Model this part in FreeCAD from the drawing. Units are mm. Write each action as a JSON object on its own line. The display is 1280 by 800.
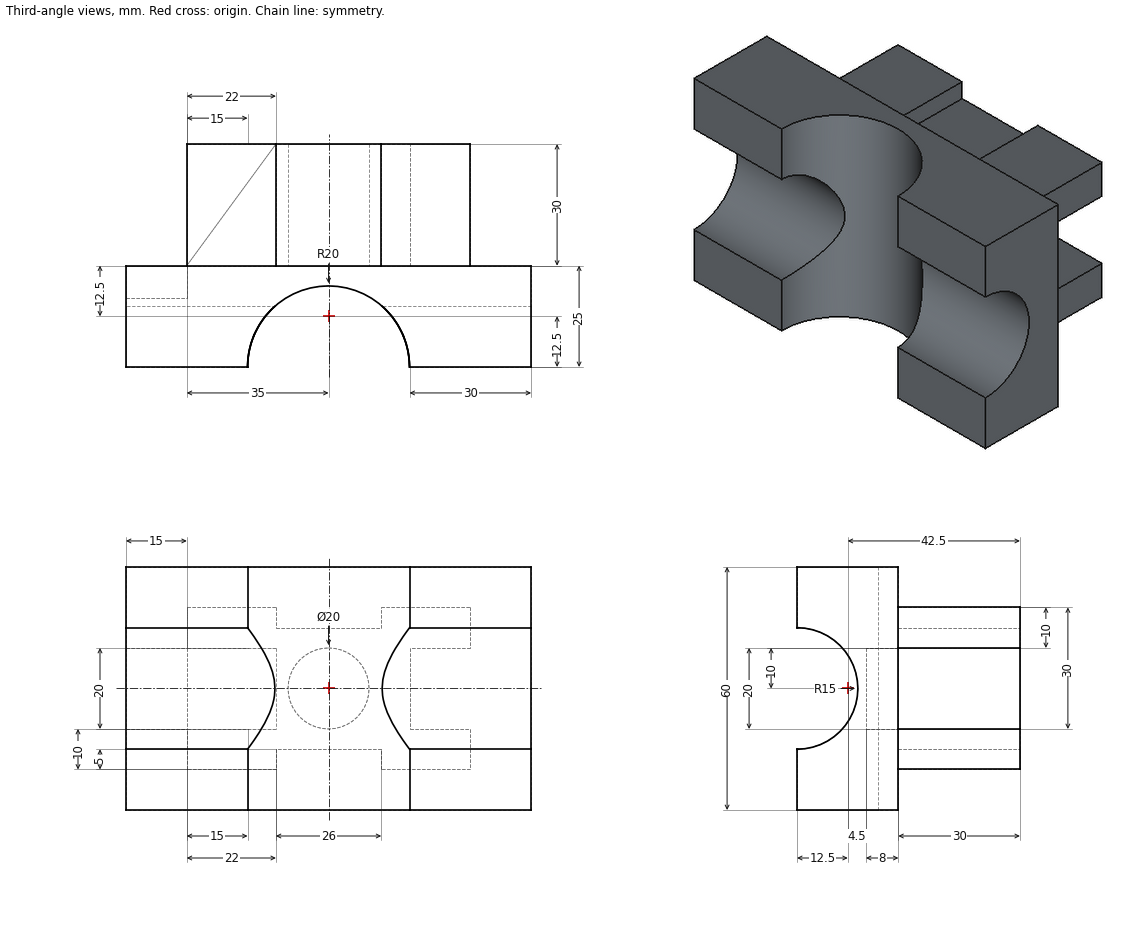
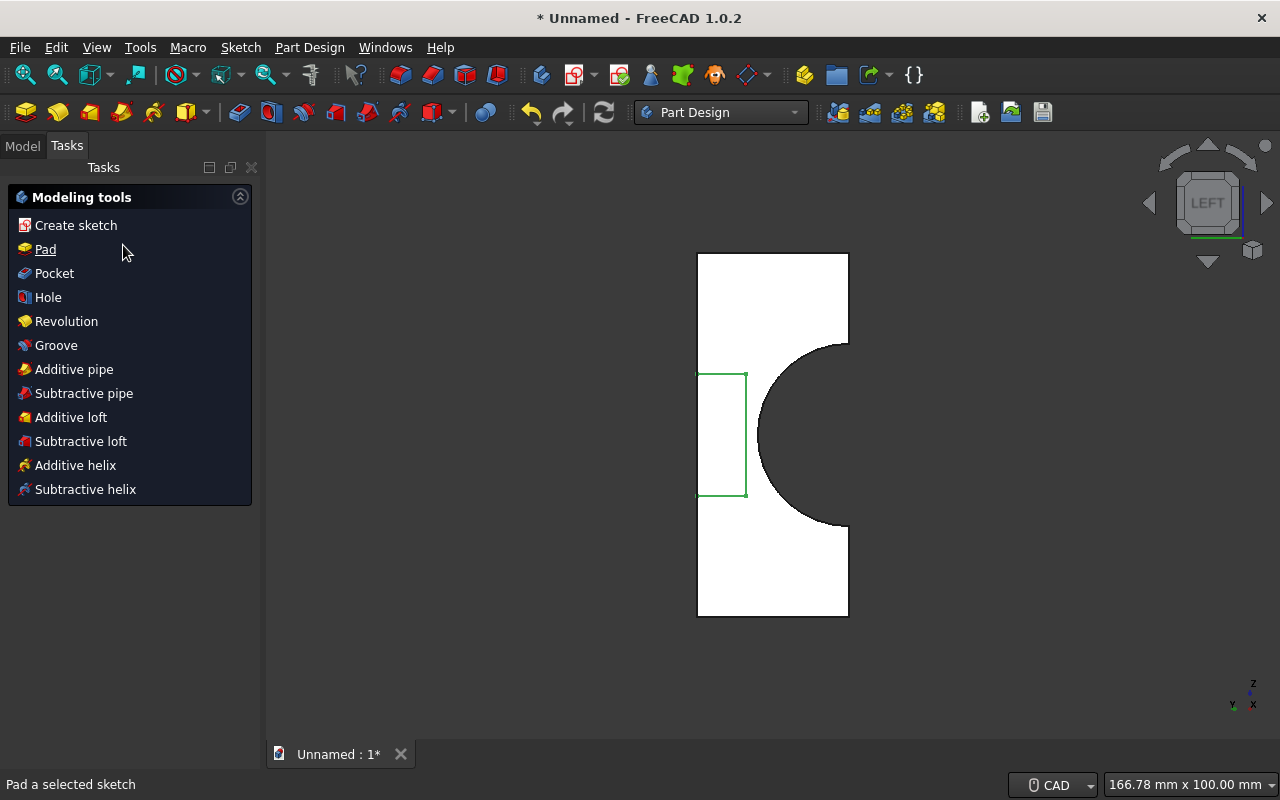
{"action": "left_click", "coordinate": [240, 112]}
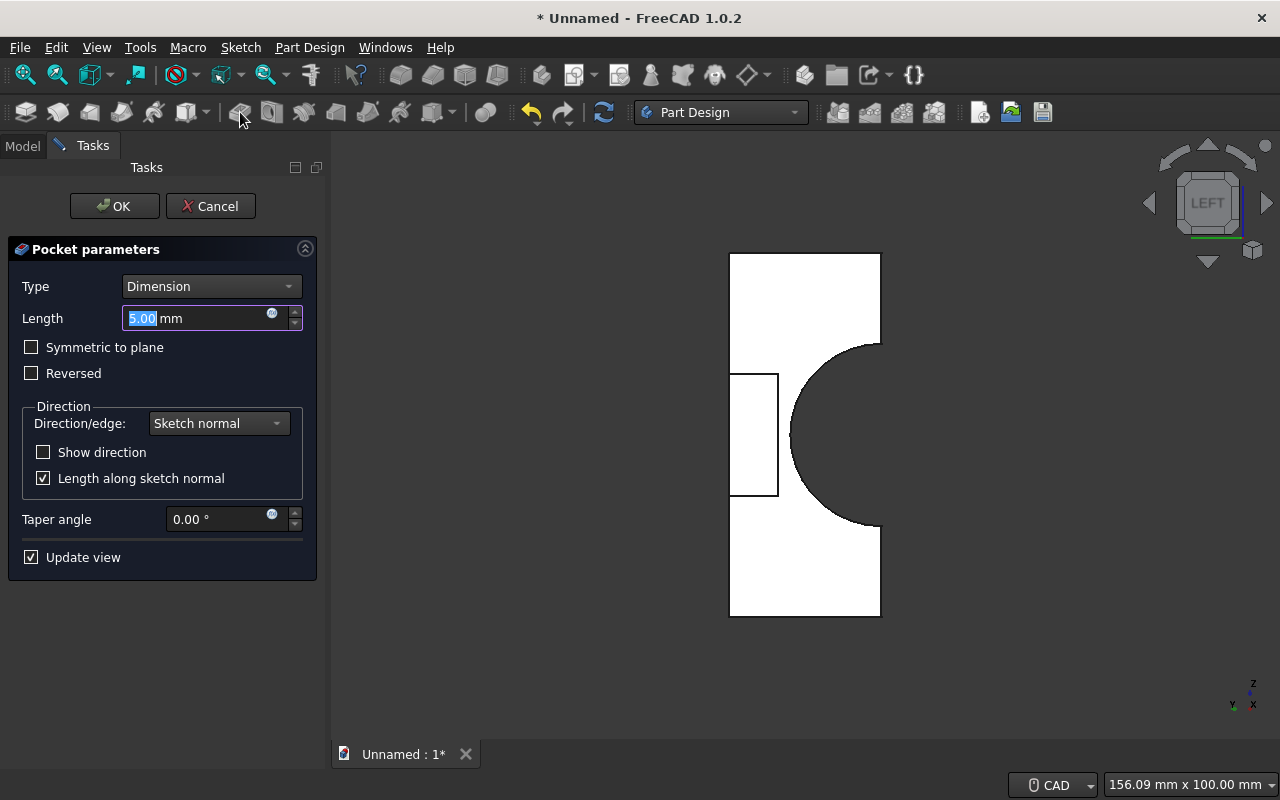
{"action": "type", "text": "15"}
{"action": "key", "text": "Tab"}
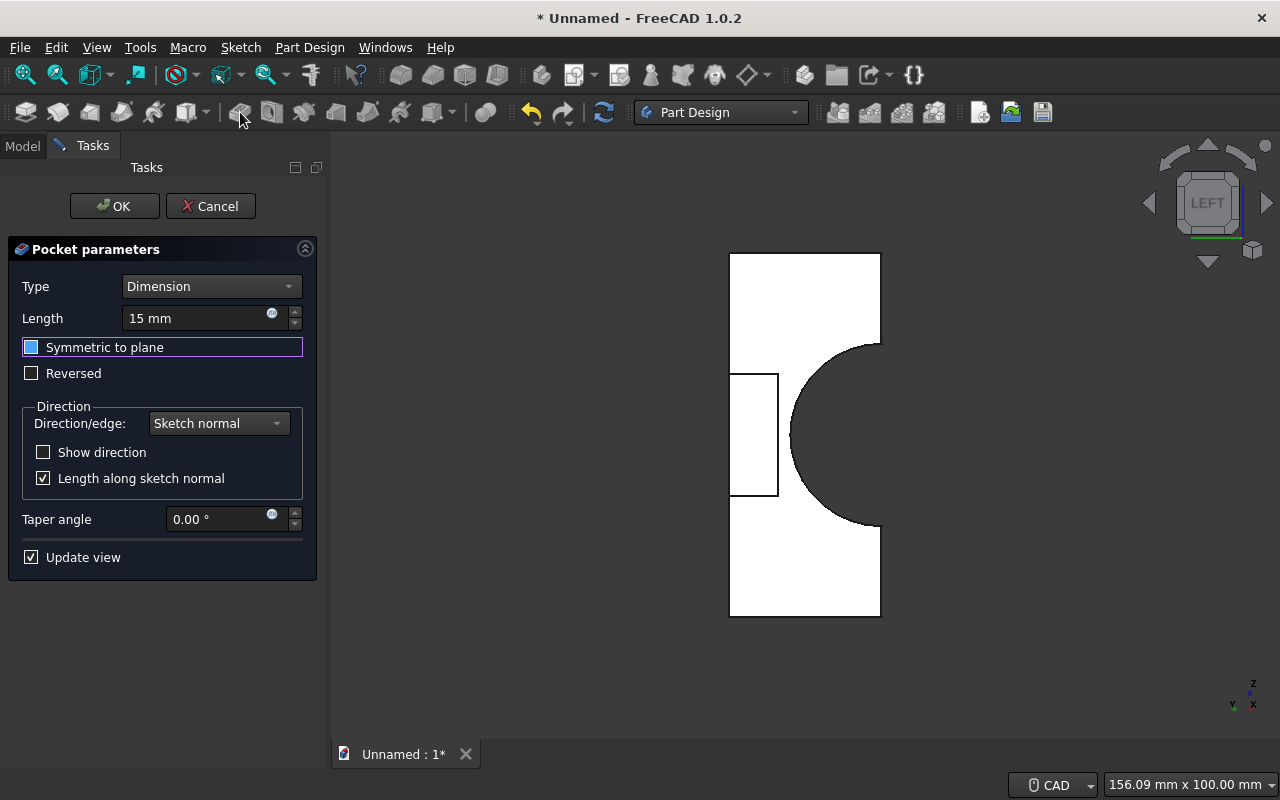
{"action": "left_click", "coordinate": [115, 206]}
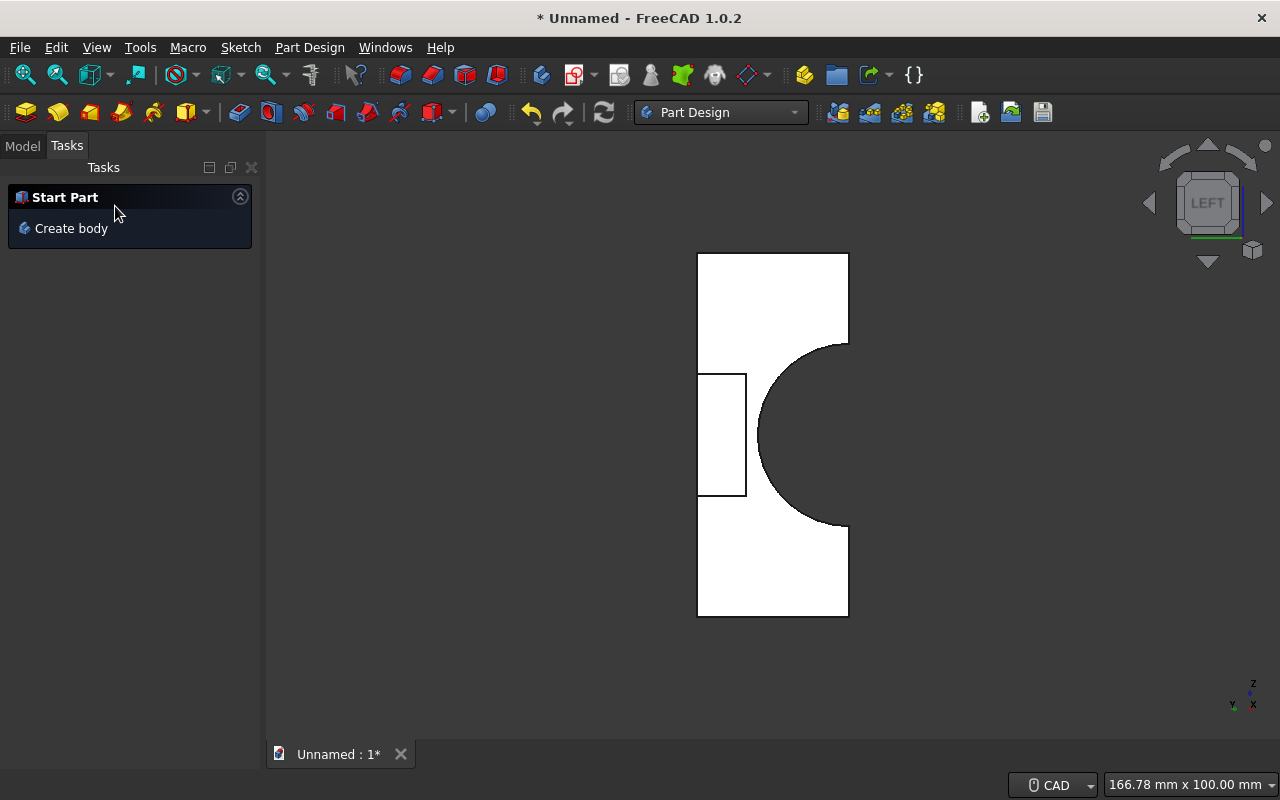
{"action": "key", "text": "4"}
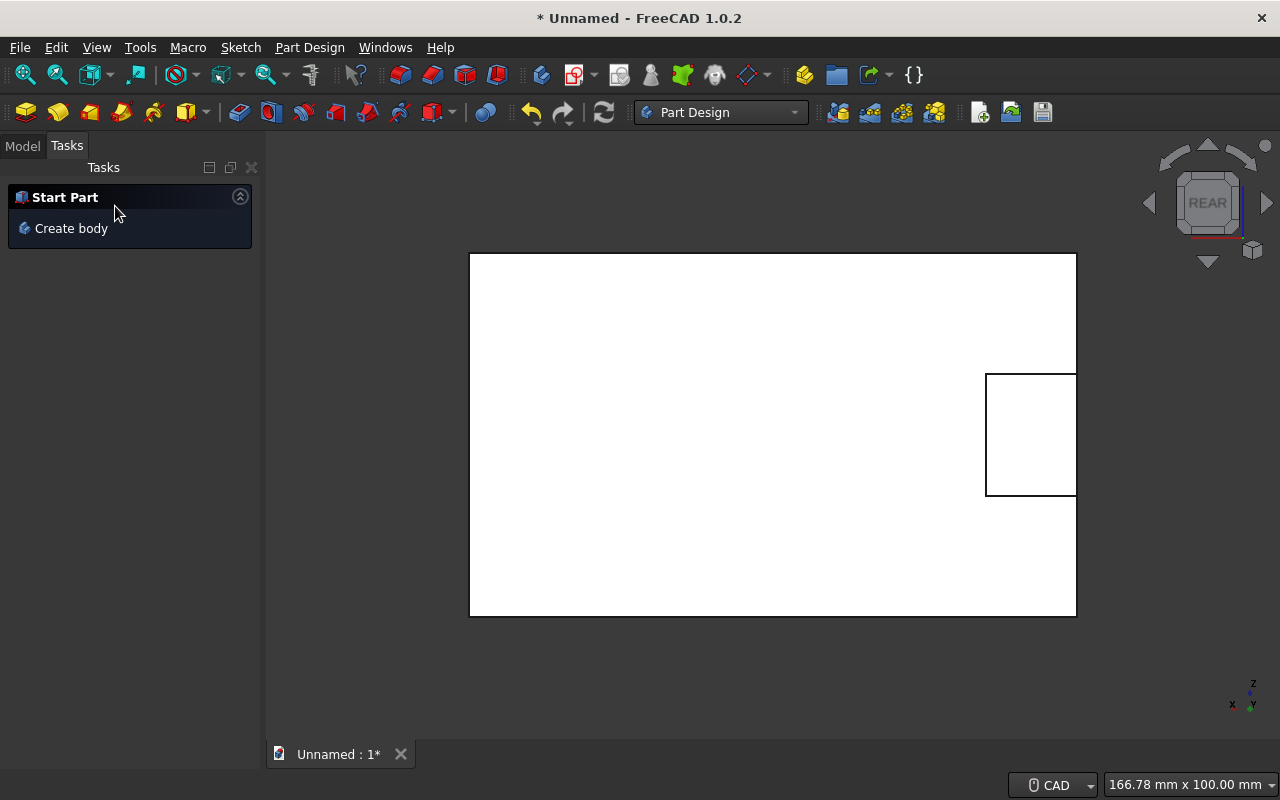
{"action": "left_click", "coordinate": [686, 434]}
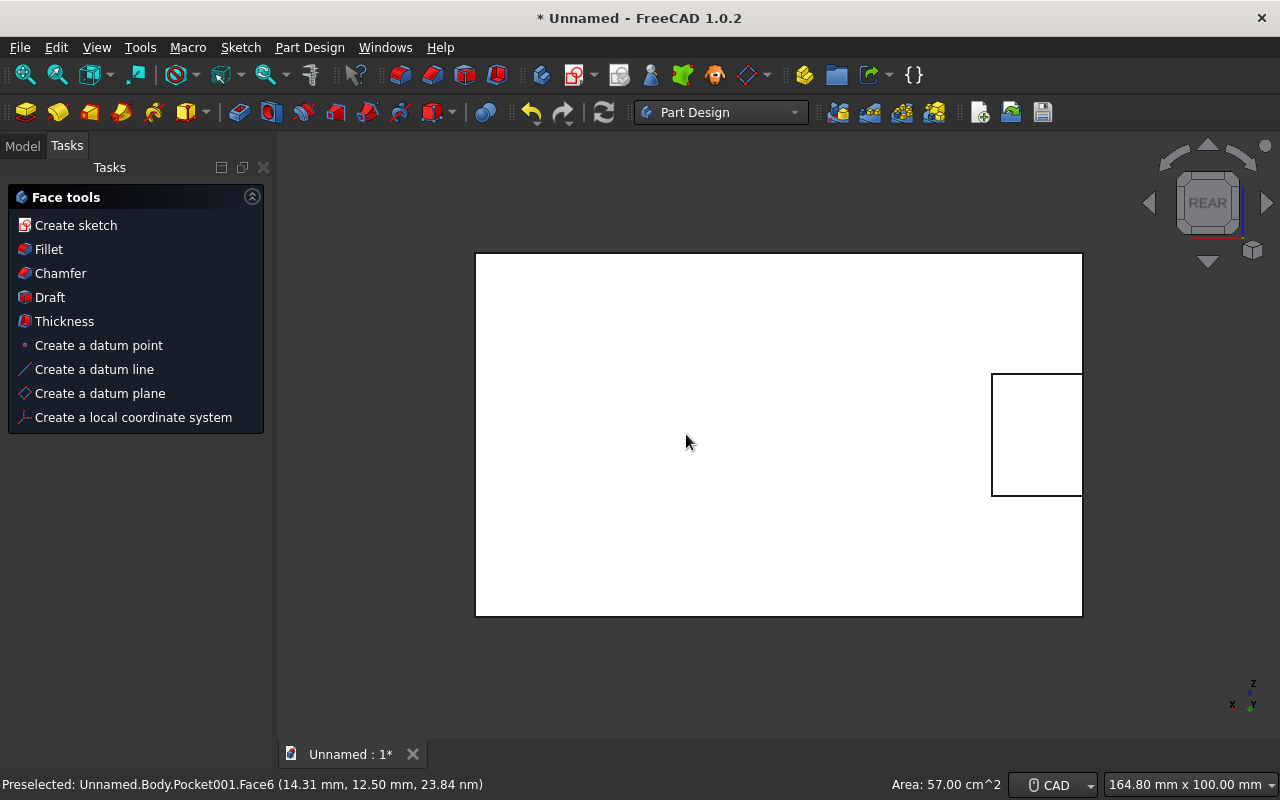
{"action": "left_click", "coordinate": [574, 76]}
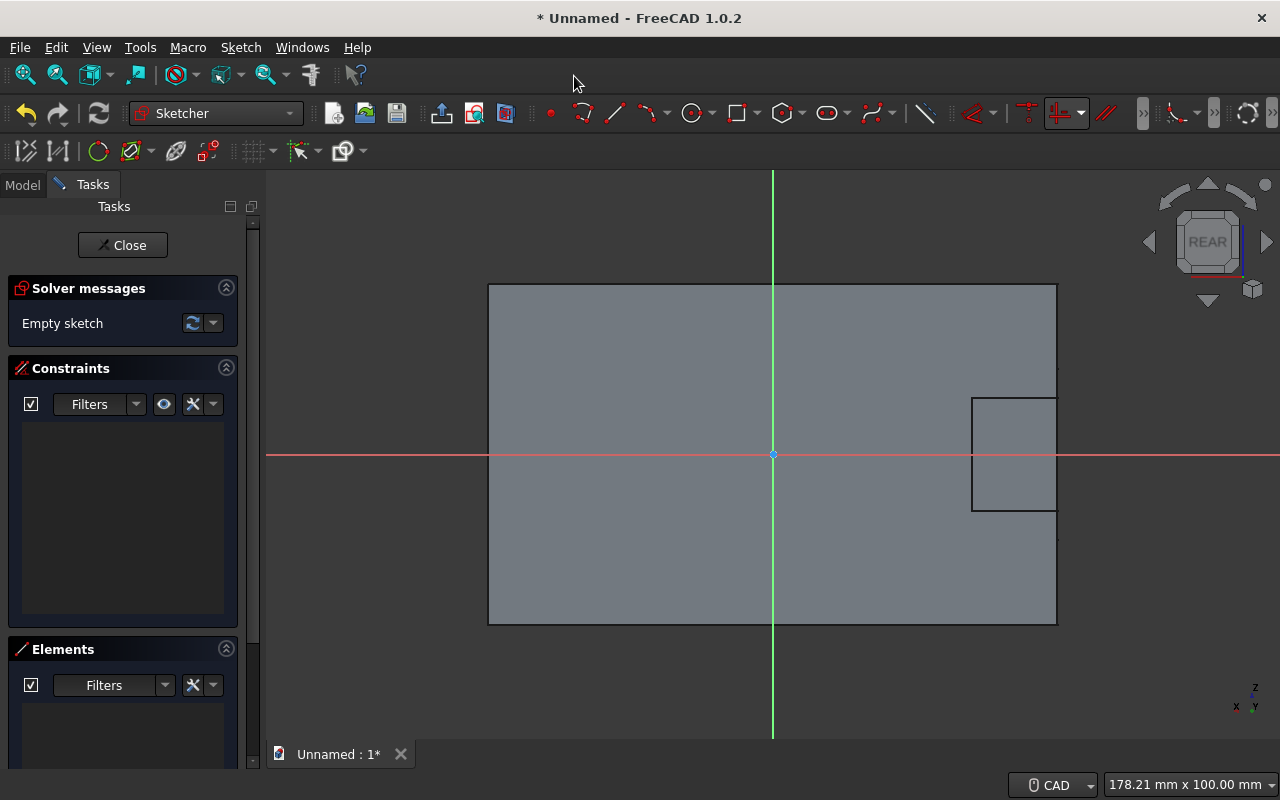
{"action": "scroll", "coordinate": [912, 455], "scroll_direction": "up", "scroll_amount": 2}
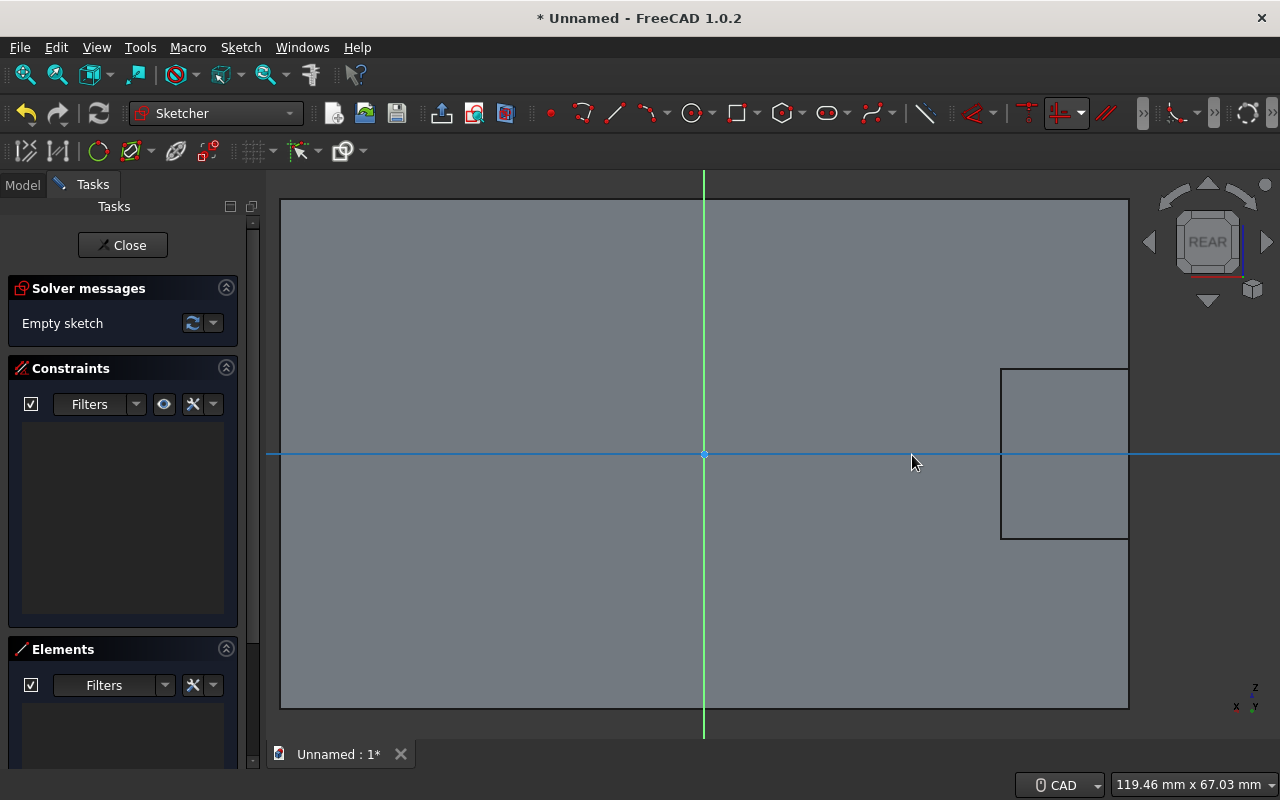
{"action": "left_click", "coordinate": [584, 114]}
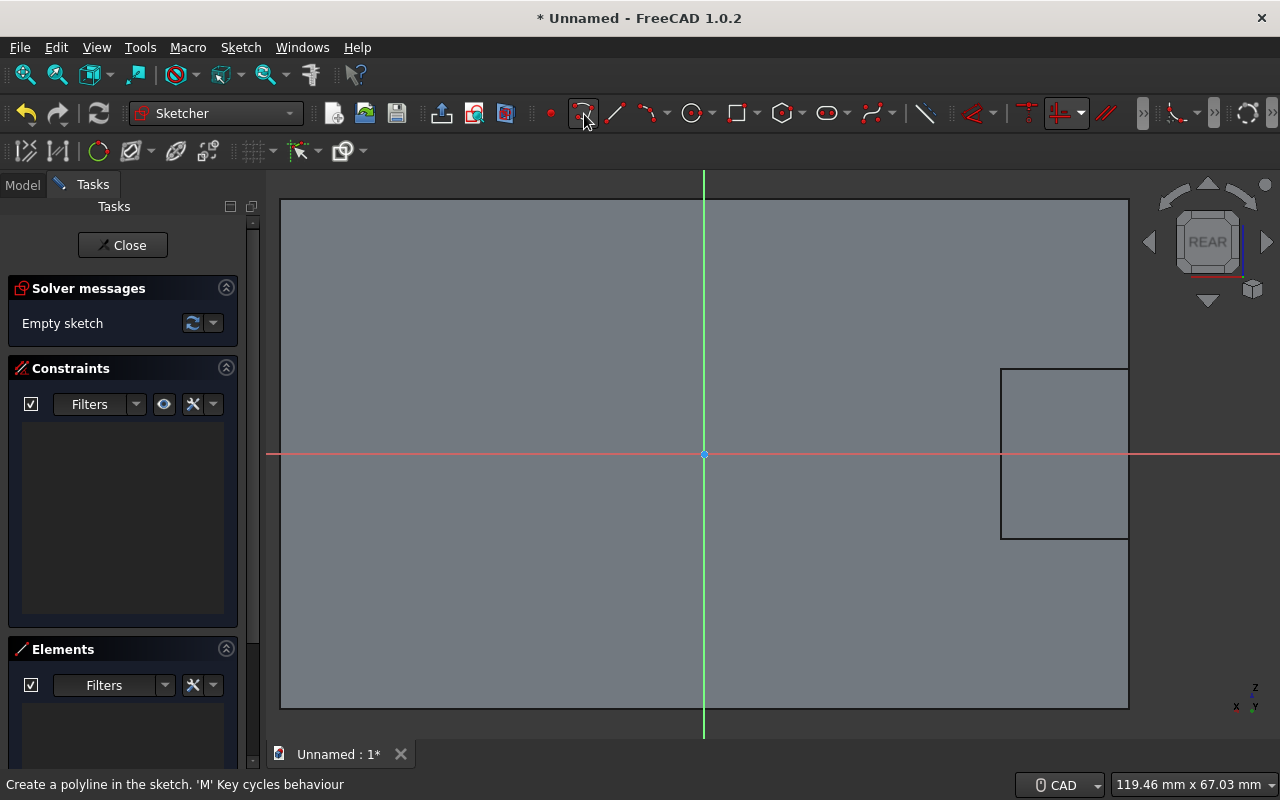
{"action": "left_click", "coordinate": [594, 581]}
{"action": "left_click", "coordinate": [815, 581]}
{"action": "left_click", "coordinate": [815, 624]}
{"action": "left_click", "coordinate": [1001, 624]}
{"action": "left_click", "coordinate": [1001, 539]}
{"action": "left_click", "coordinate": [874, 539]}
{"action": "left_click", "coordinate": [874, 369]}
{"action": "left_click", "coordinate": [1001, 369]}
{"action": "left_click", "coordinate": [1001, 284]}
{"action": "left_click", "coordinate": [815, 284]}
{"action": "left_click", "coordinate": [815, 327]}
{"action": "left_click", "coordinate": [594, 327]}
{"action": "left_click", "coordinate": [594, 284]}
{"action": "left_click", "coordinate": [407, 284]}
{"action": "left_click", "coordinate": [407, 369]}
{"action": "left_click", "coordinate": [535, 369]}
{"action": "left_click", "coordinate": [535, 539]}
{"action": "left_click", "coordinate": [407, 539]}
{"action": "left_click", "coordinate": [407, 624]}
{"action": "left_click", "coordinate": [594, 624]}
{"action": "left_click", "coordinate": [594, 582]}